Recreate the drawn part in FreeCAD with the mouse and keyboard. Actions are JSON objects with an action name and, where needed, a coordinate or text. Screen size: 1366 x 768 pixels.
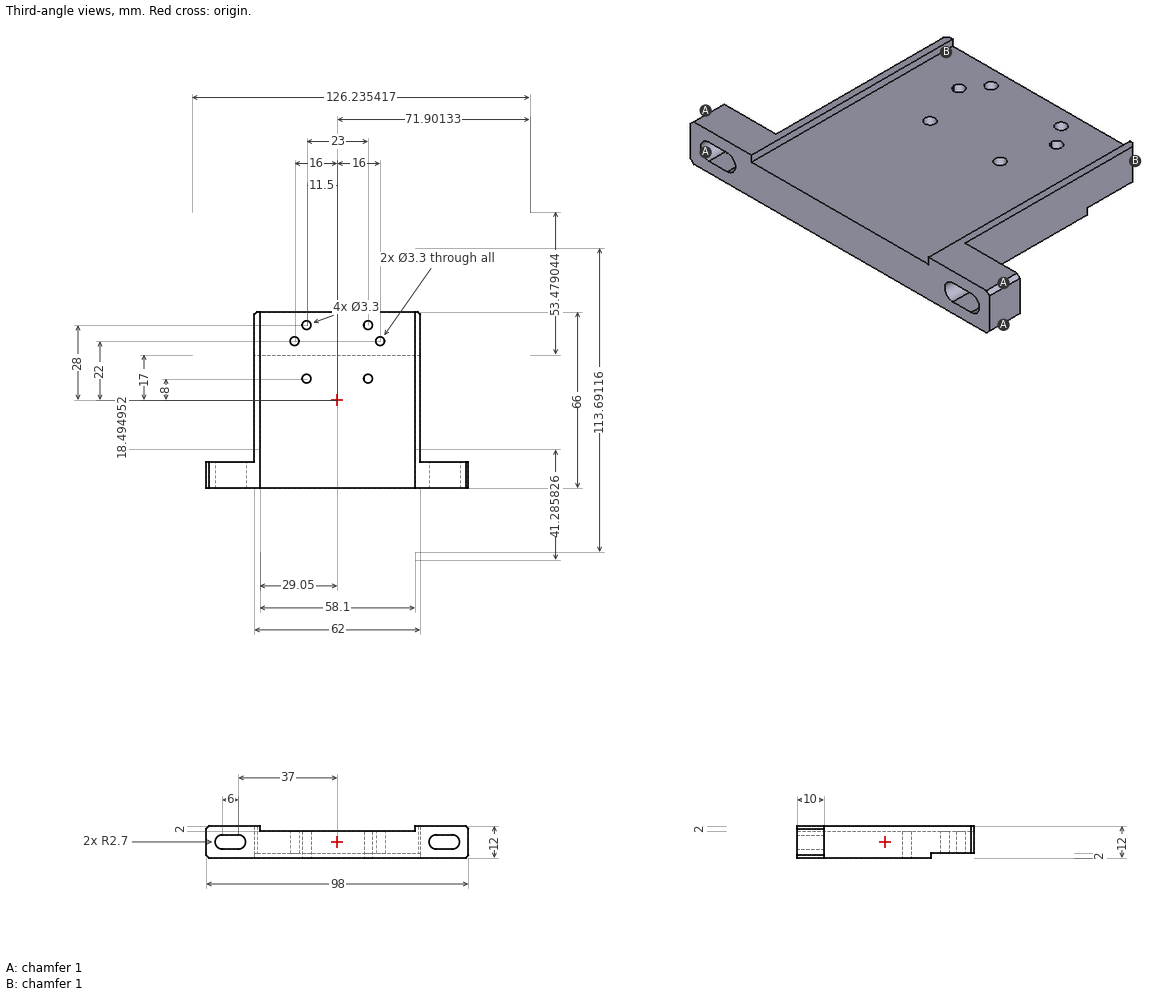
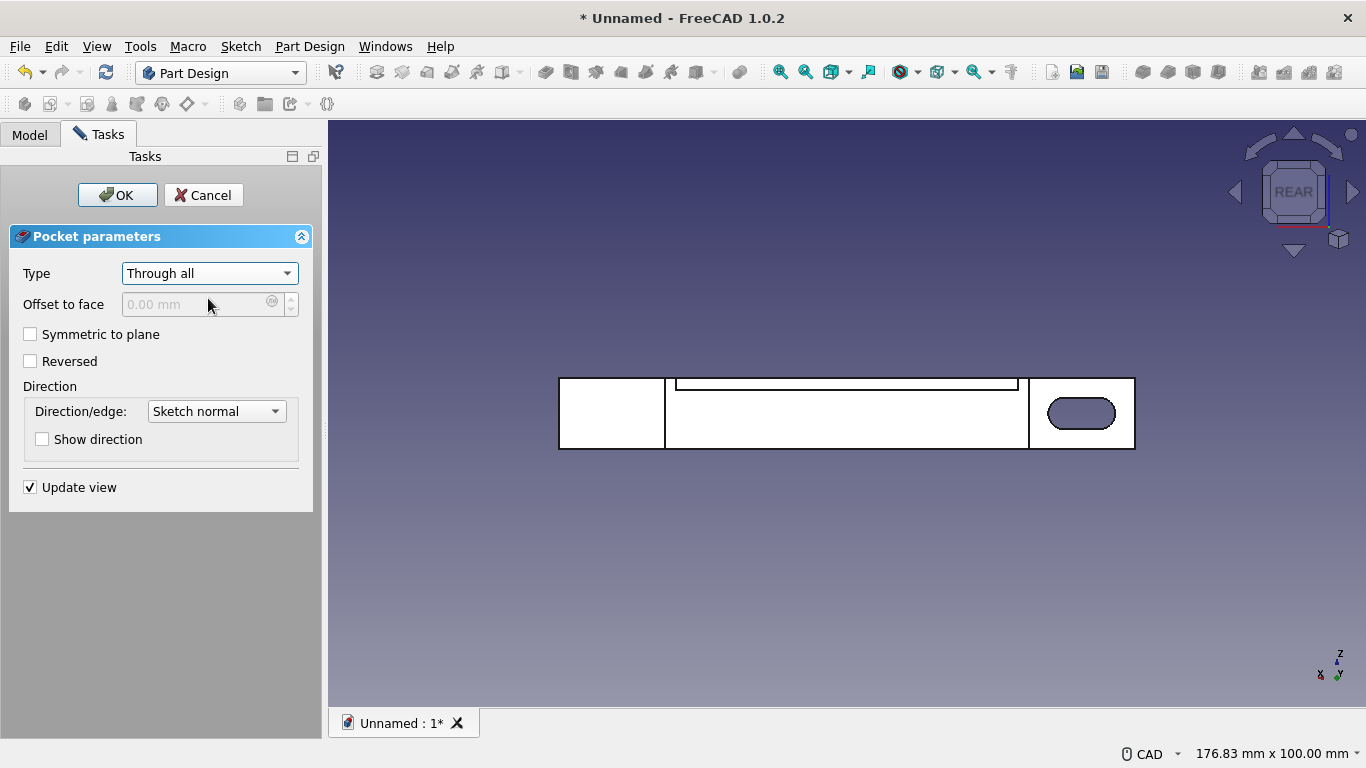
{"action": "left_click", "coordinate": [118, 195]}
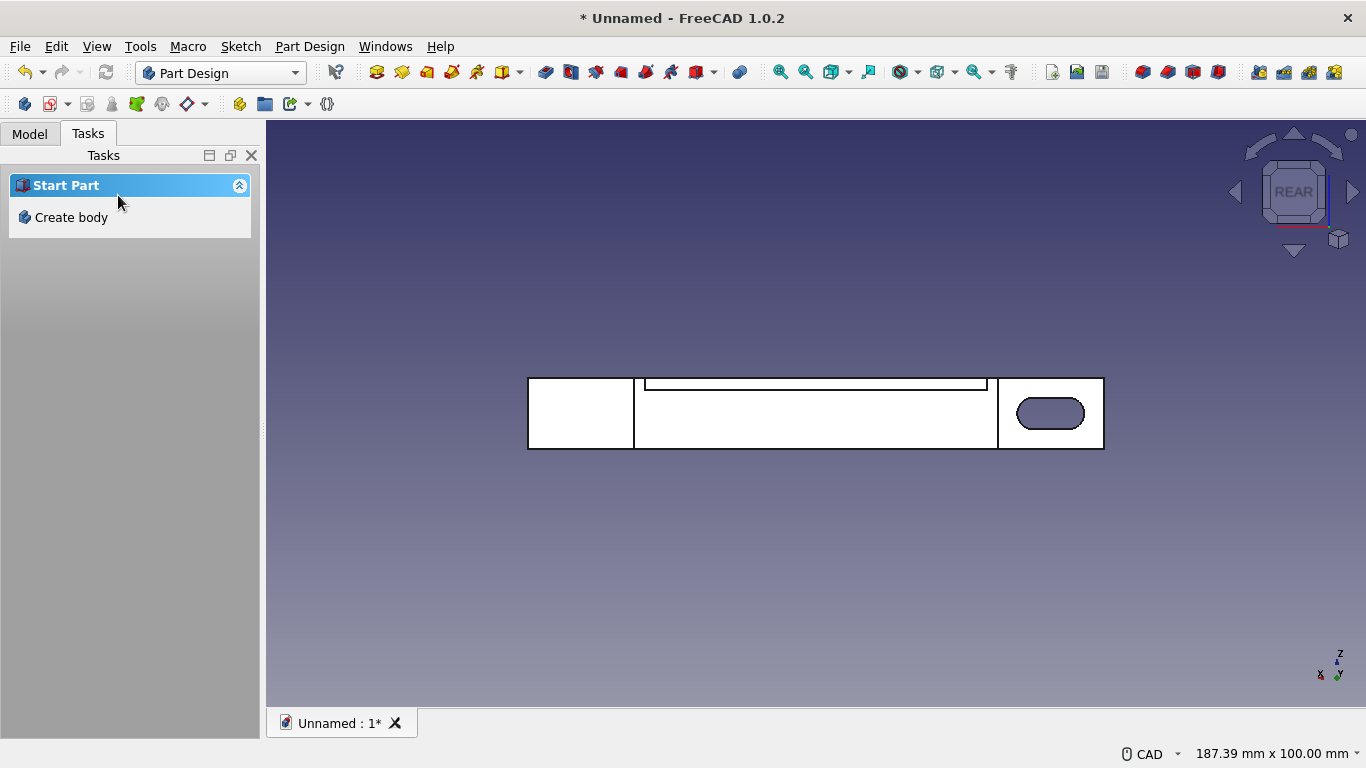
{"action": "left_click", "coordinate": [30, 134]}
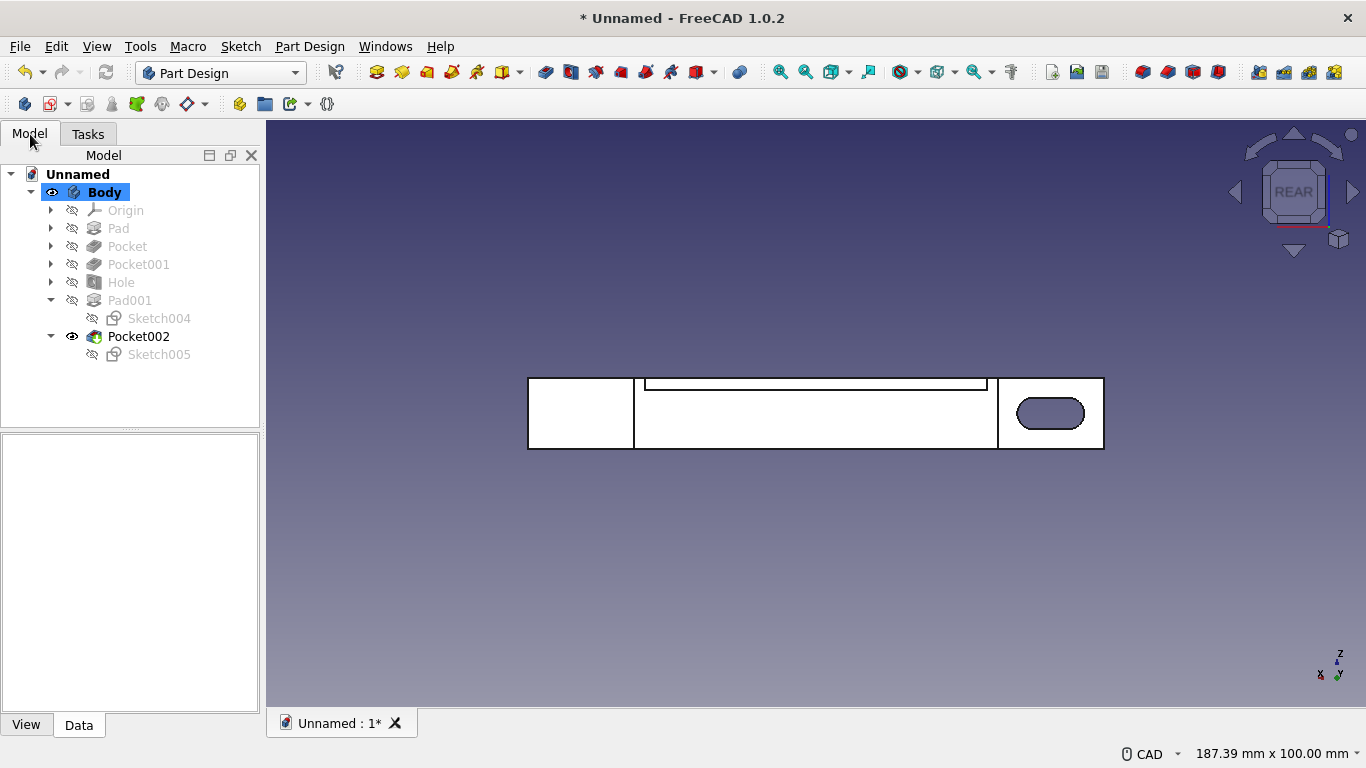
{"action": "left_click", "coordinate": [117, 336]}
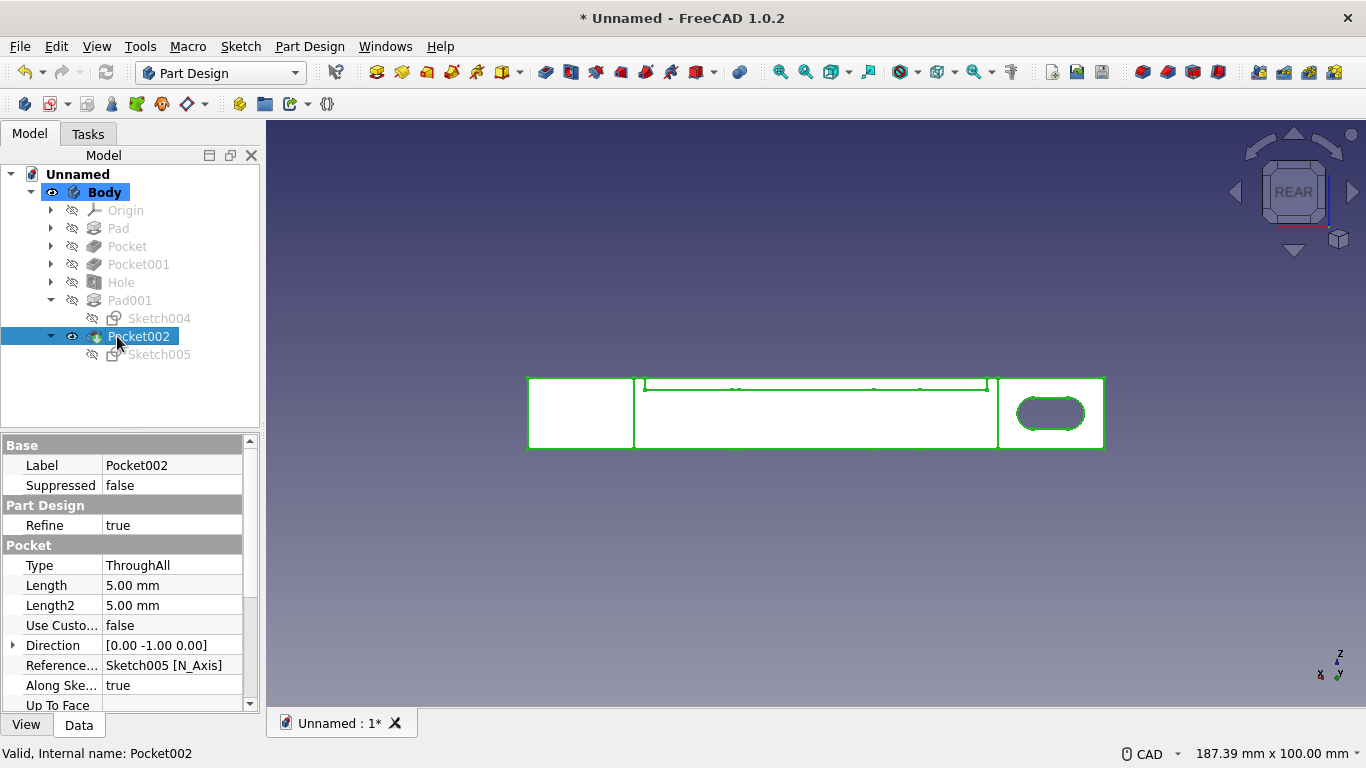
{"action": "left_click", "coordinate": [1259, 72]}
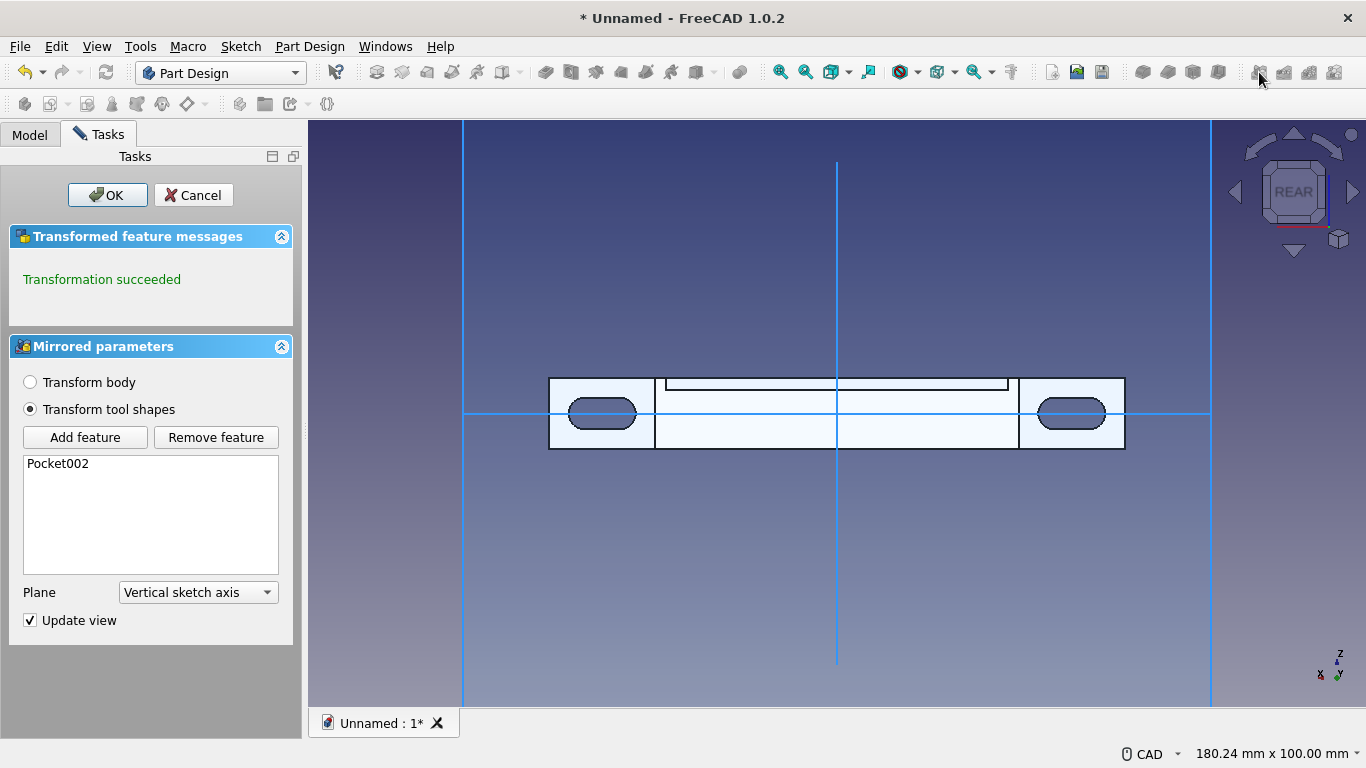
{"action": "left_click", "coordinate": [199, 592]}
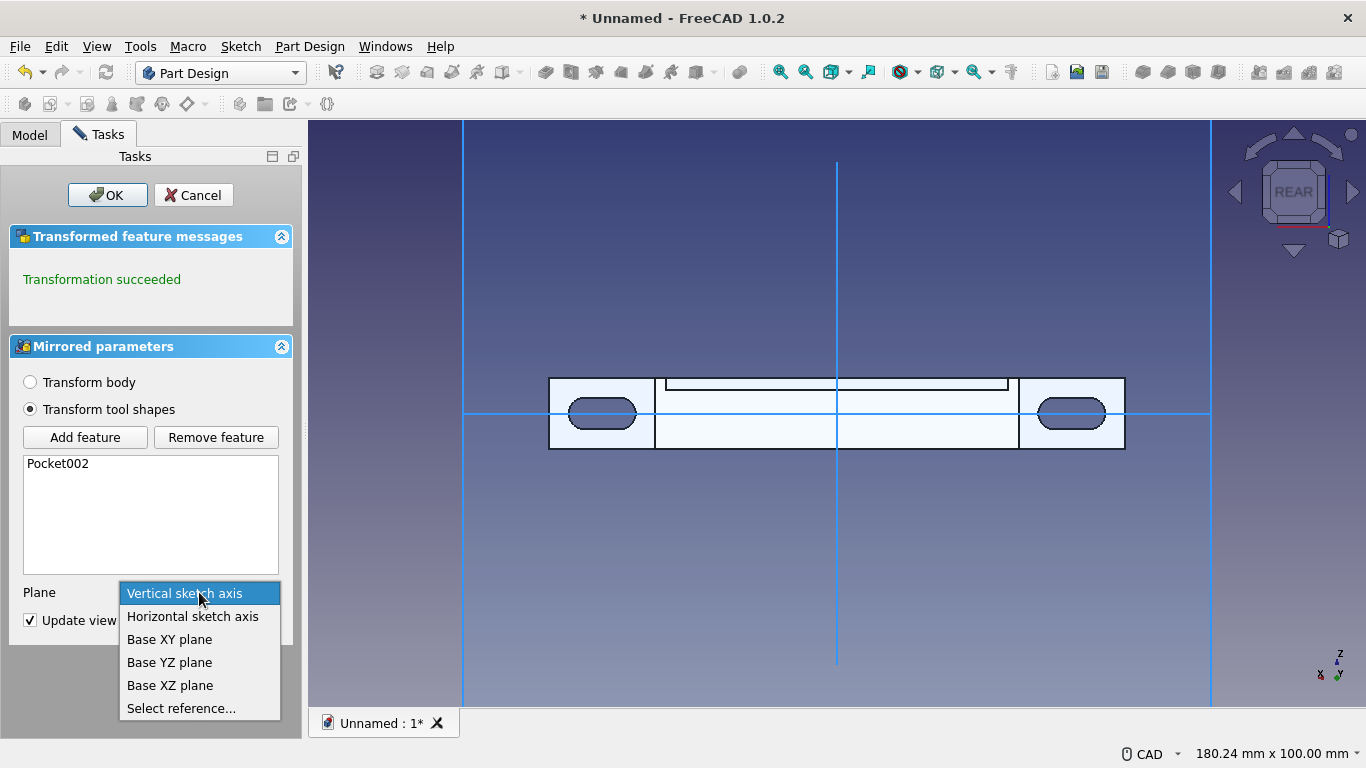
{"action": "left_click", "coordinate": [198, 662]}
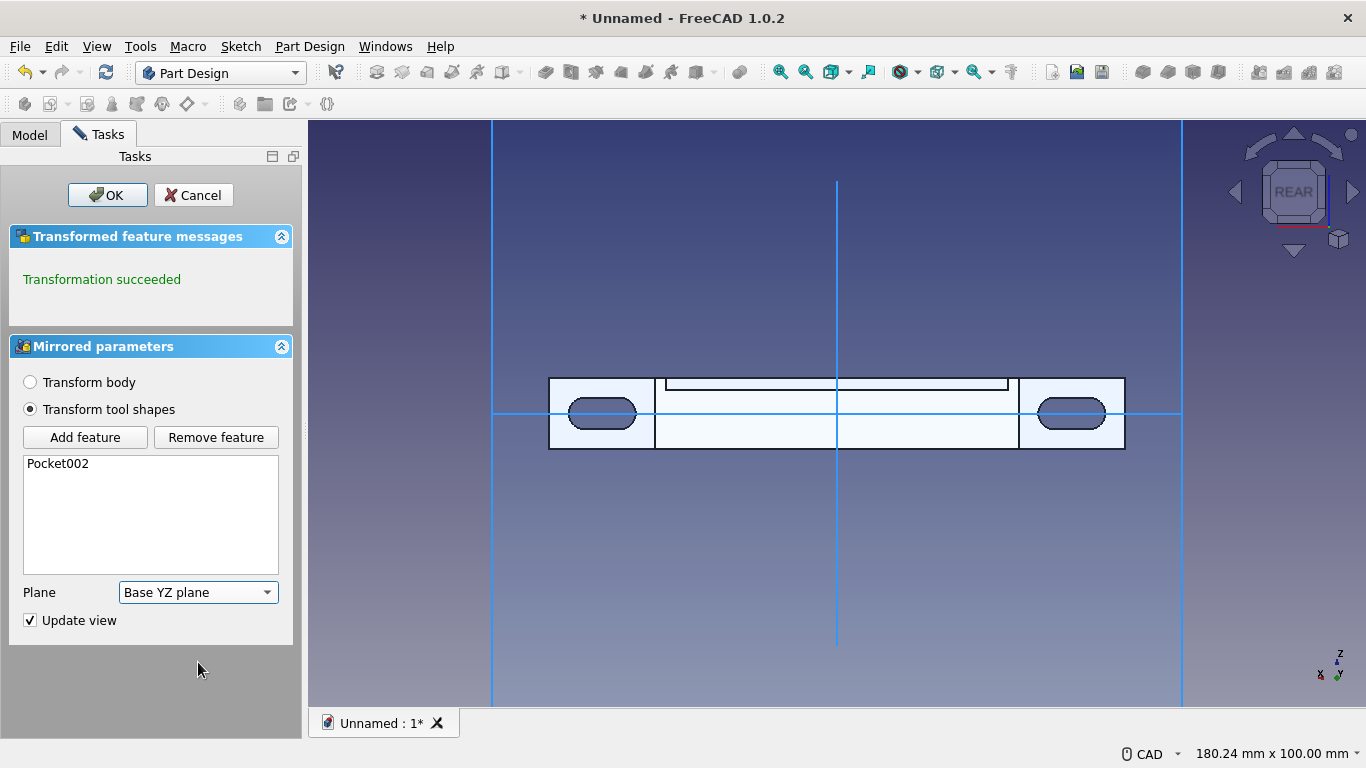
{"action": "left_click", "coordinate": [108, 195]}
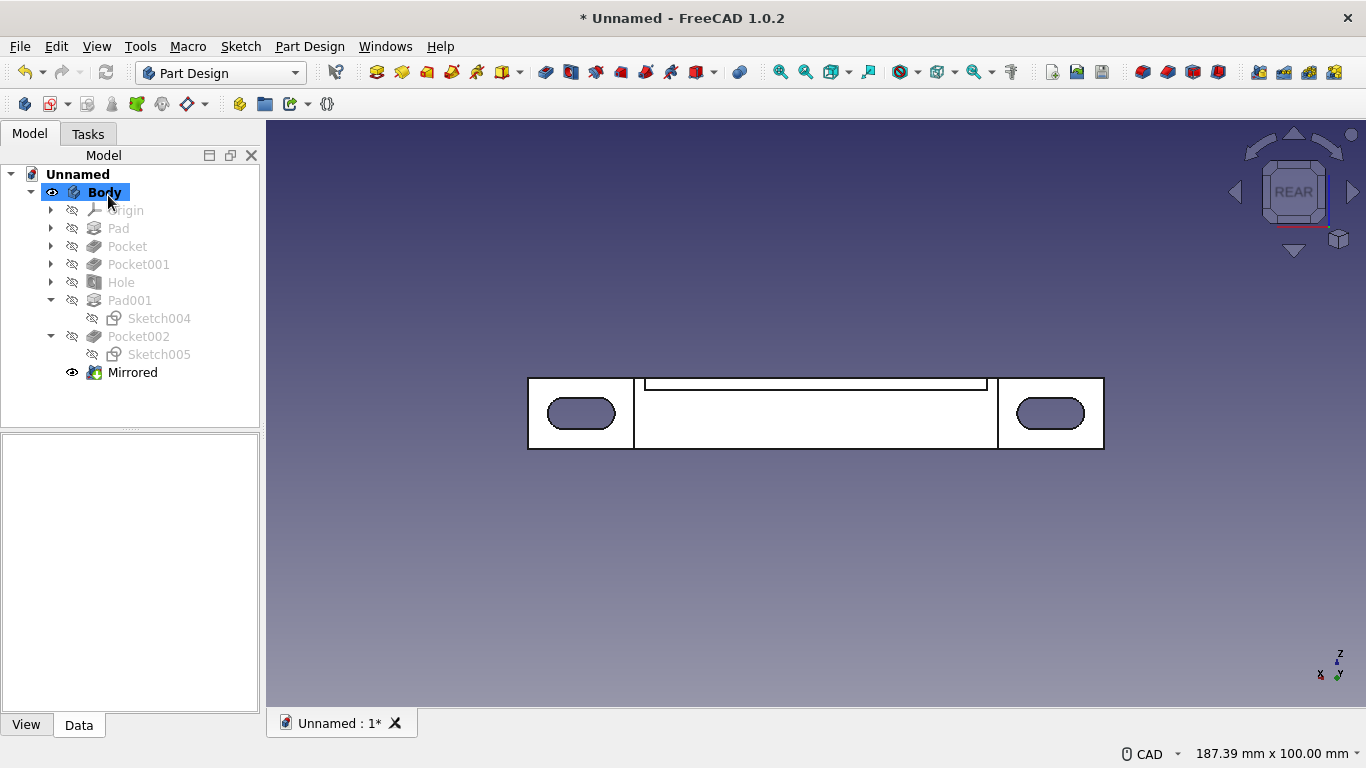
{"action": "key", "text": "0"}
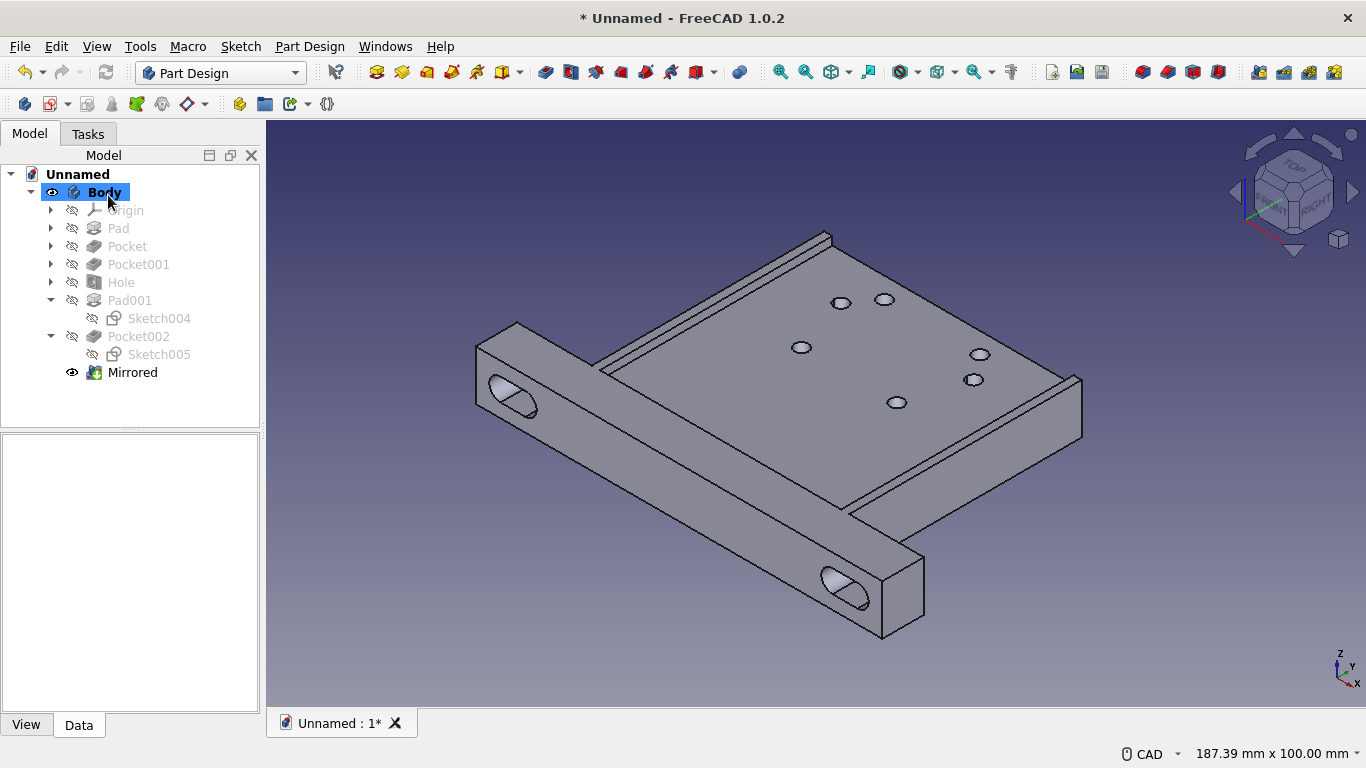
{"action": "left_click", "coordinate": [873, 552]}